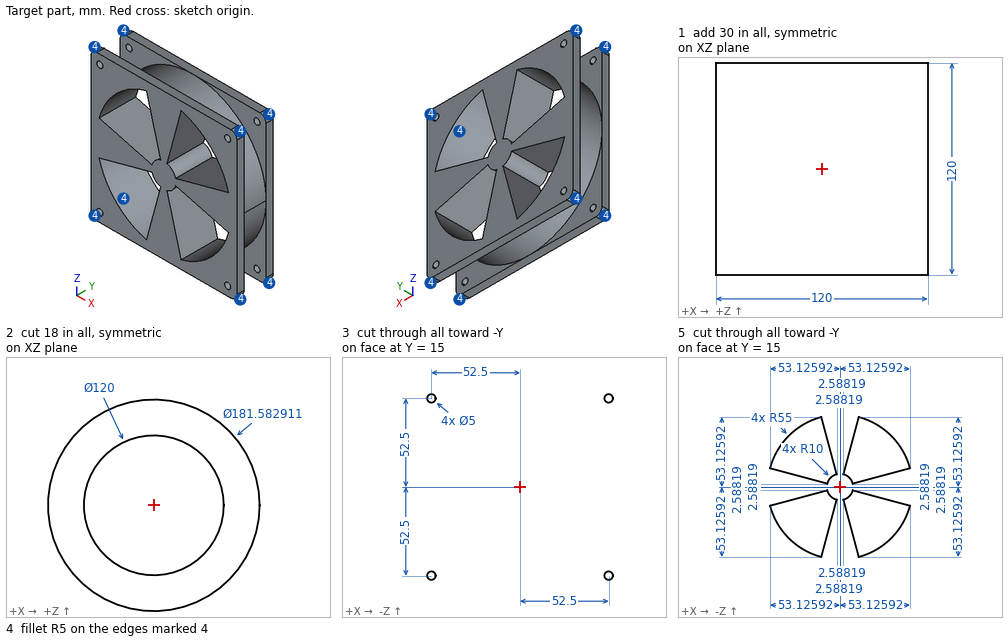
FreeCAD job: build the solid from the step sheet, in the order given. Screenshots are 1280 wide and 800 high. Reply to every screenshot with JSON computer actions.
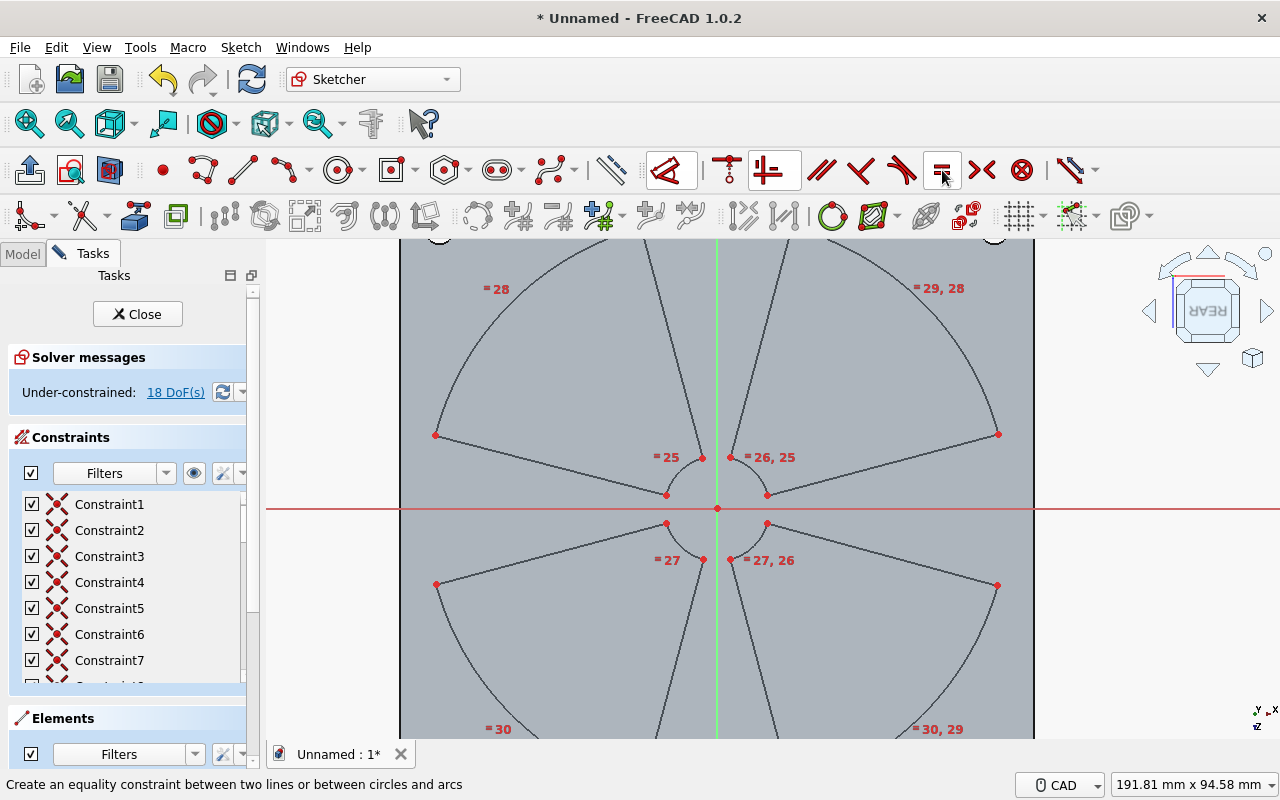
{"action": "left_click", "coordinate": [472, 352]}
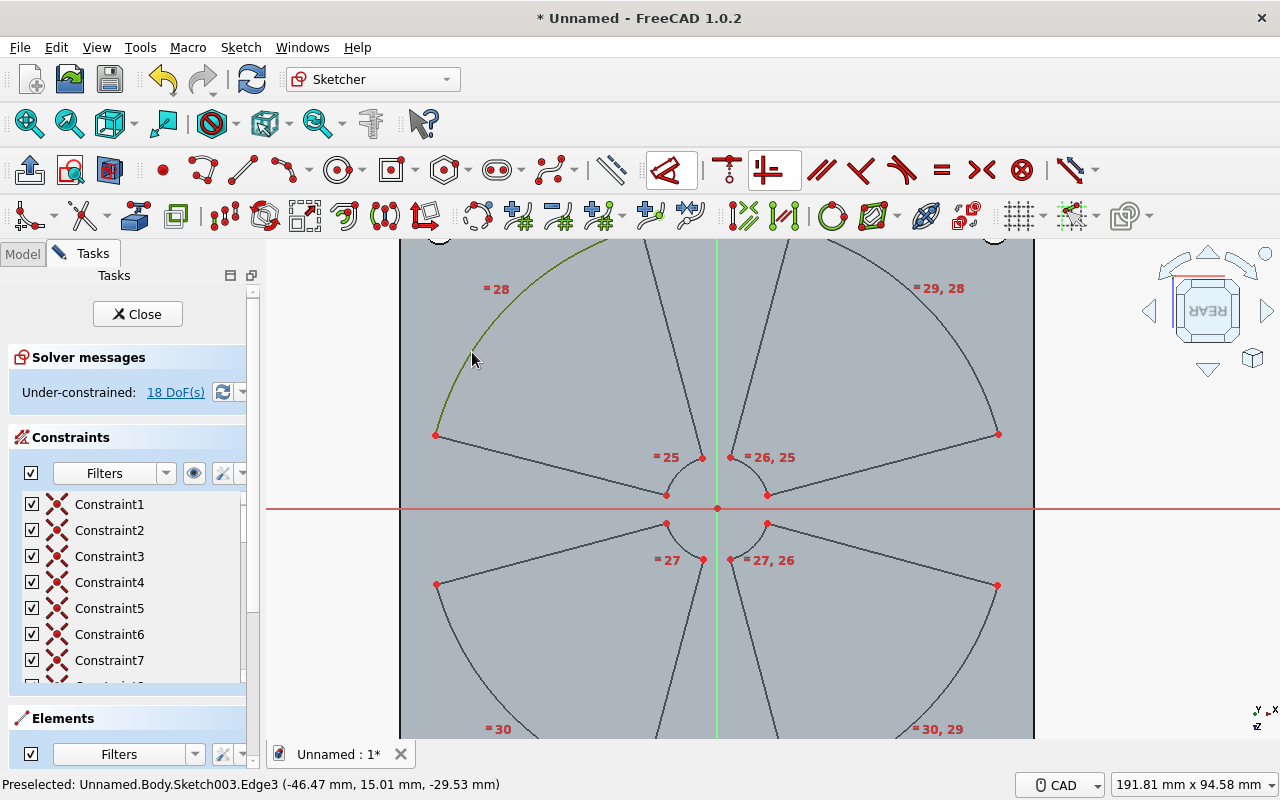
{"action": "left_click", "coordinate": [692, 170]}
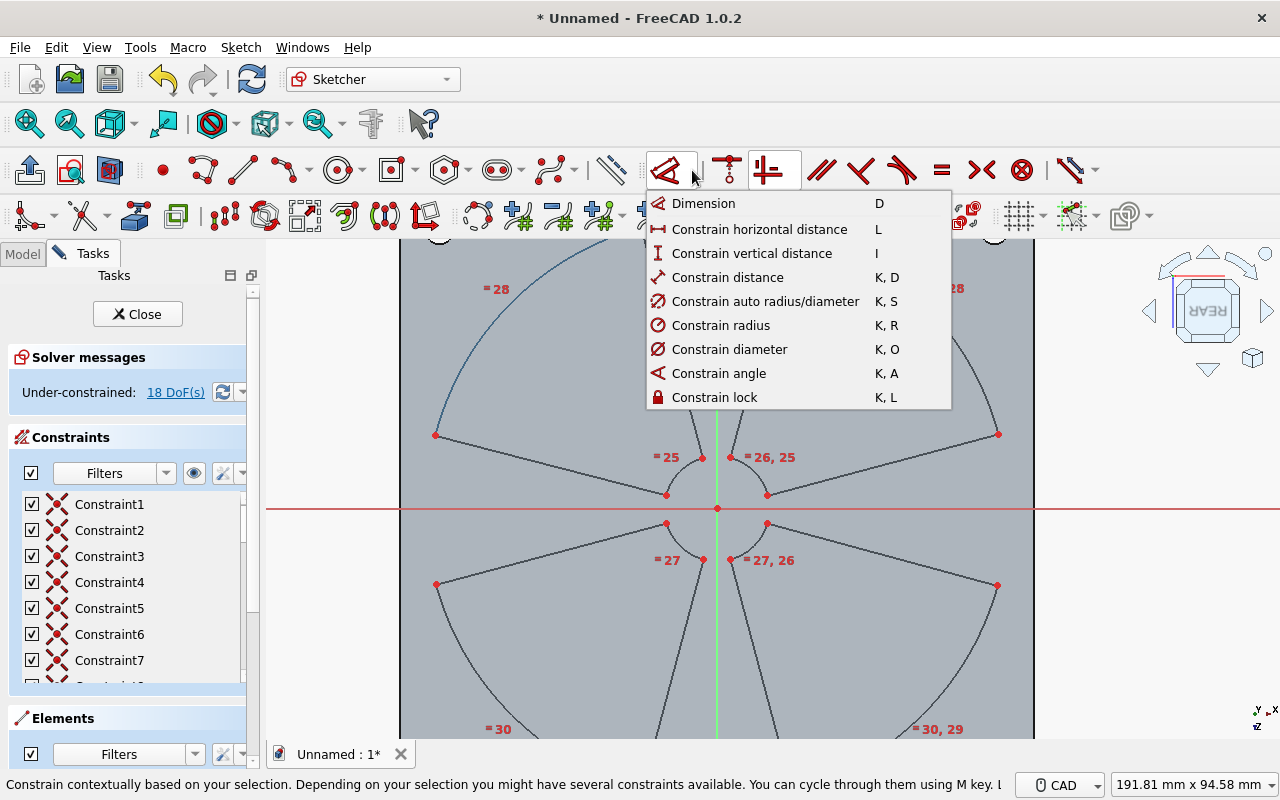
{"action": "left_click", "coordinate": [799, 325]}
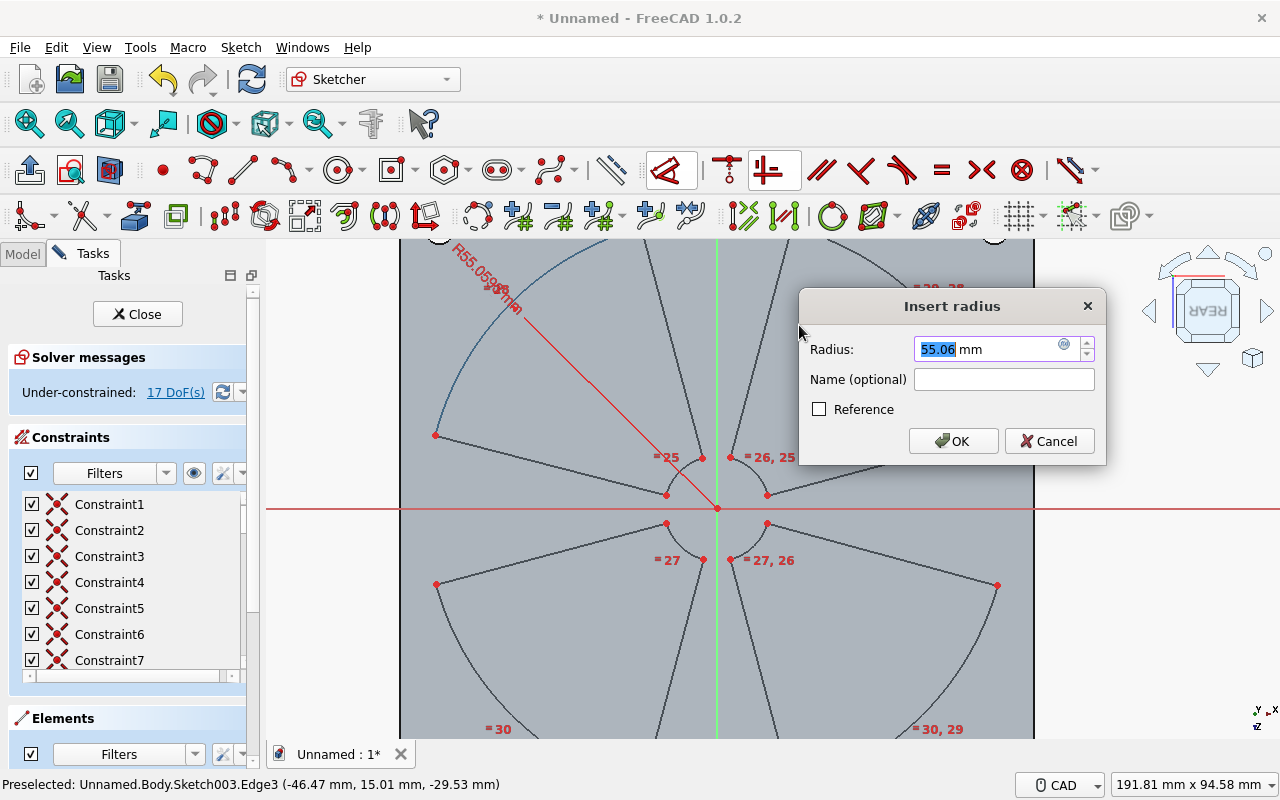
{"action": "type", "text": "55"}
{"action": "key", "text": "Return"}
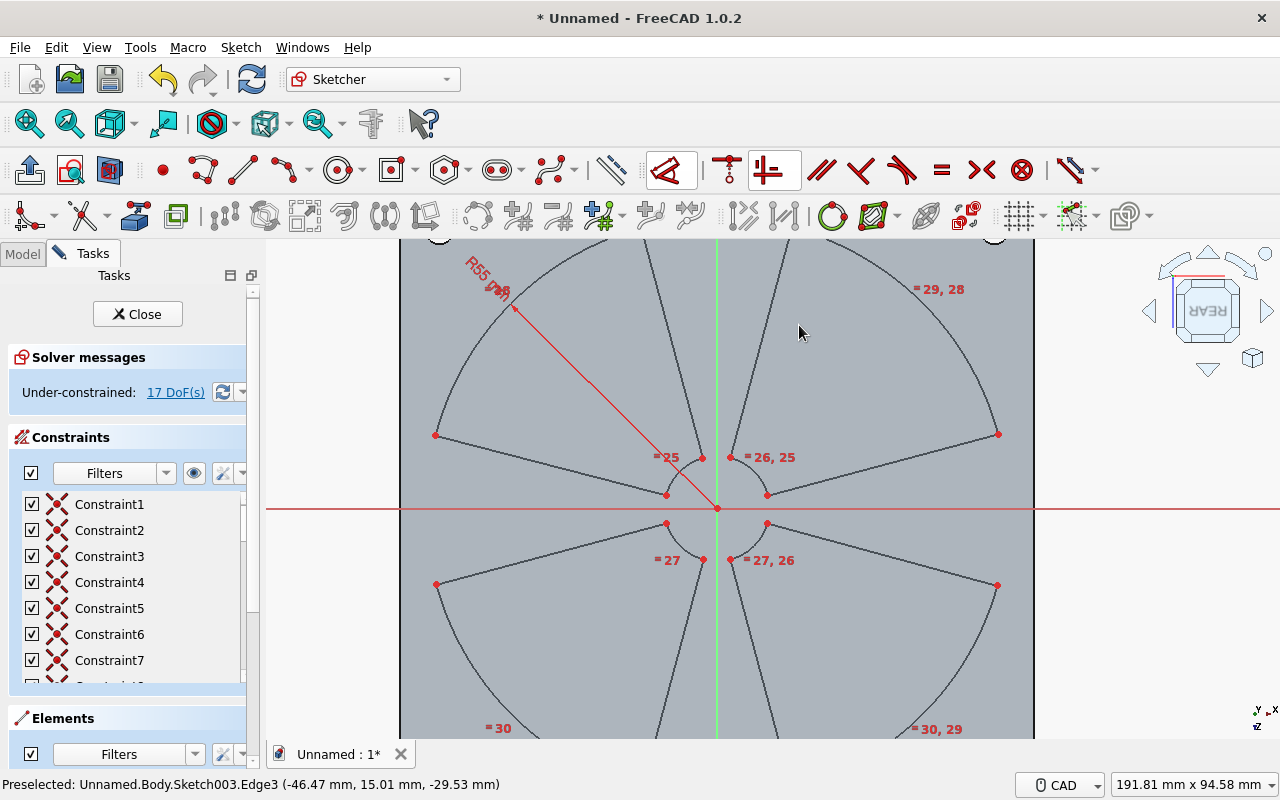
{"action": "left_click", "coordinate": [688, 465]}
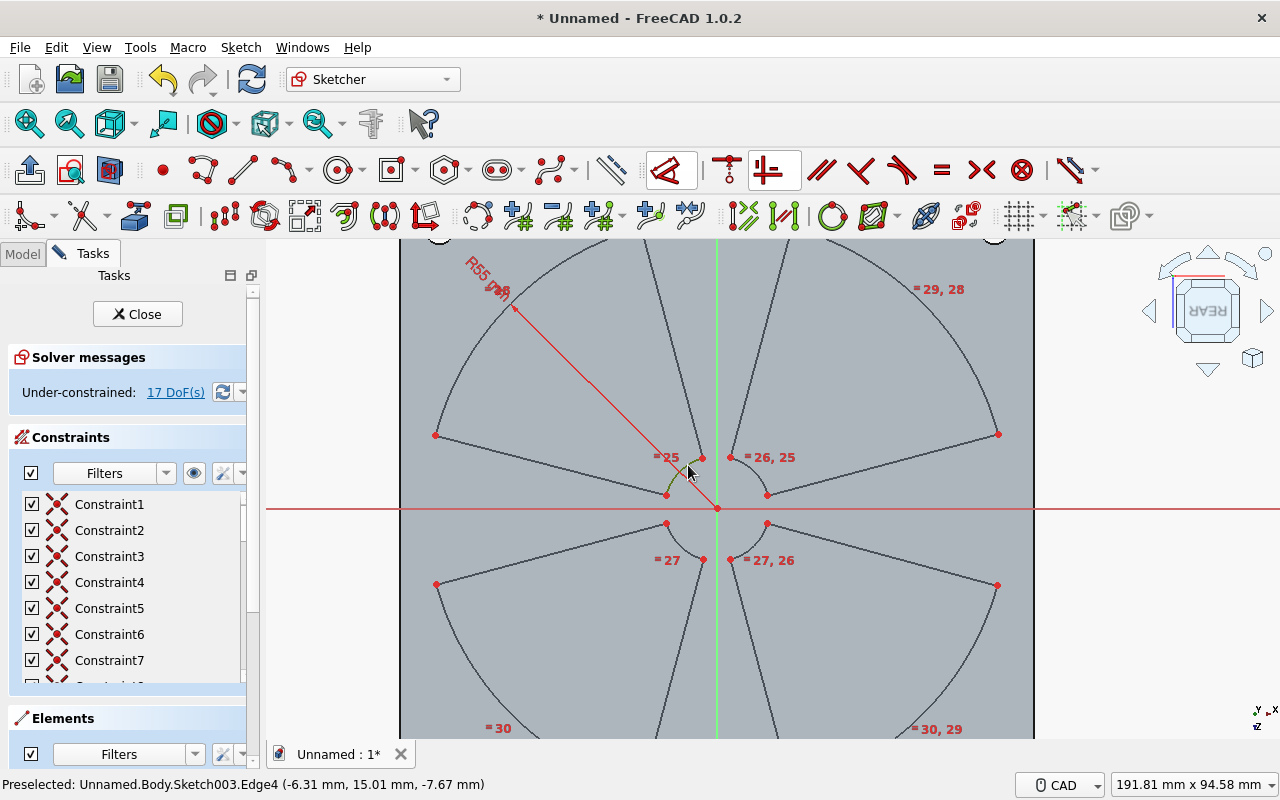
{"action": "left_click", "coordinate": [692, 170]}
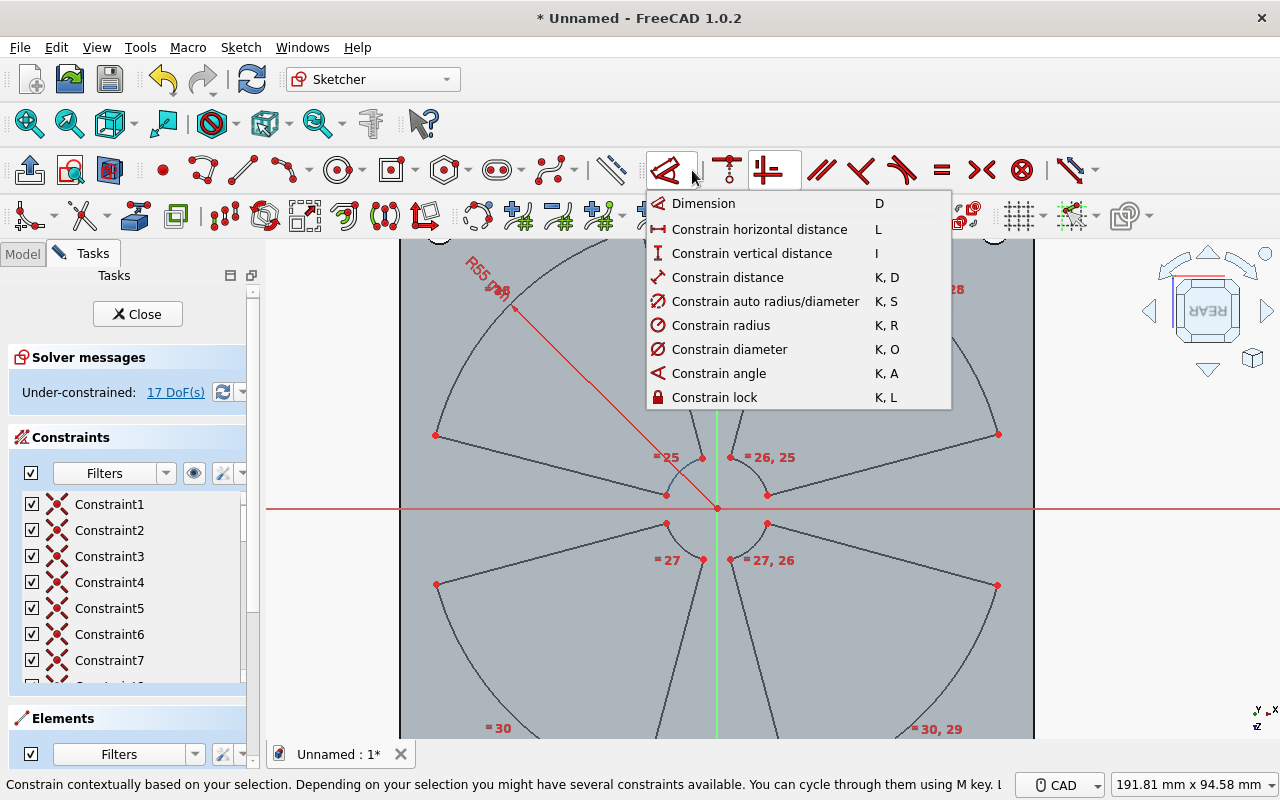
{"action": "left_click", "coordinate": [799, 325]}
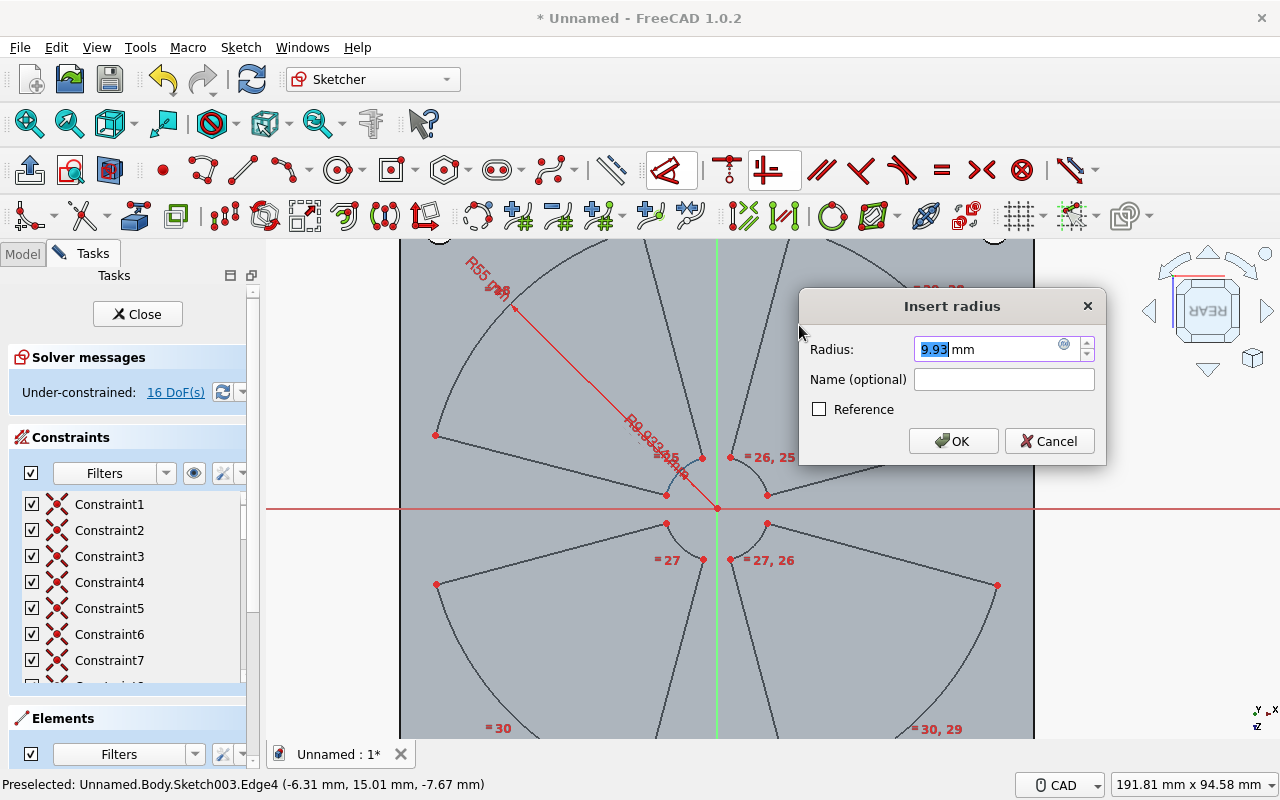
{"action": "type", "text": "10"}
{"action": "key", "text": "Return"}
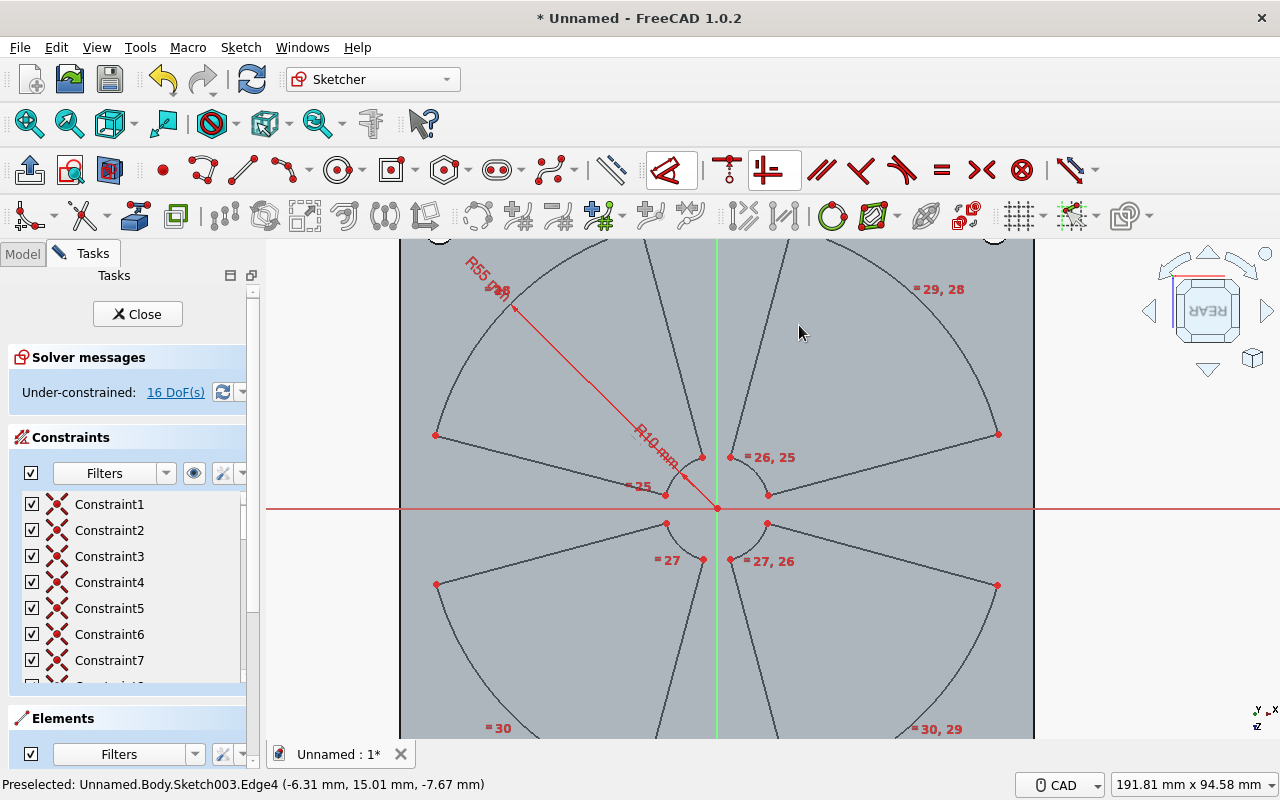
{"action": "scroll", "coordinate": [703, 458], "scroll_direction": "up", "scroll_amount": 6}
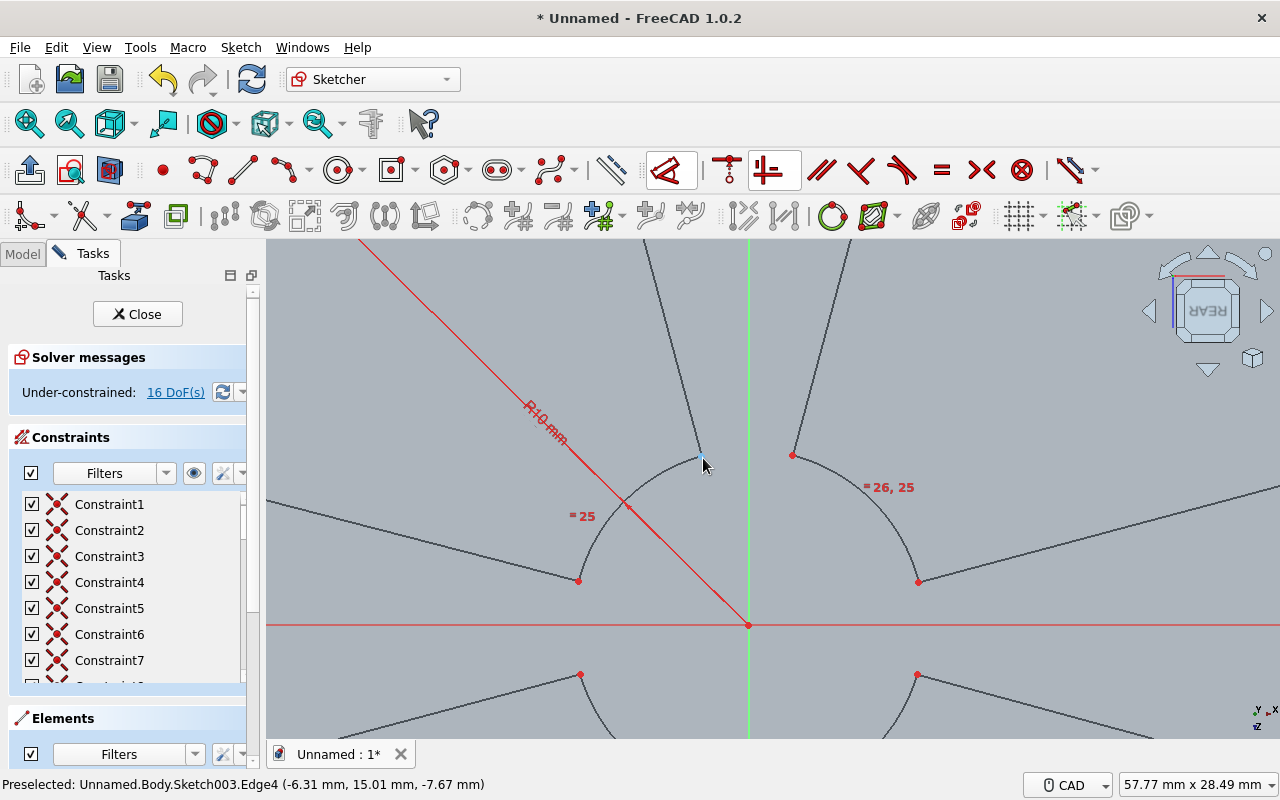
{"action": "left_click", "coordinate": [702, 456]}